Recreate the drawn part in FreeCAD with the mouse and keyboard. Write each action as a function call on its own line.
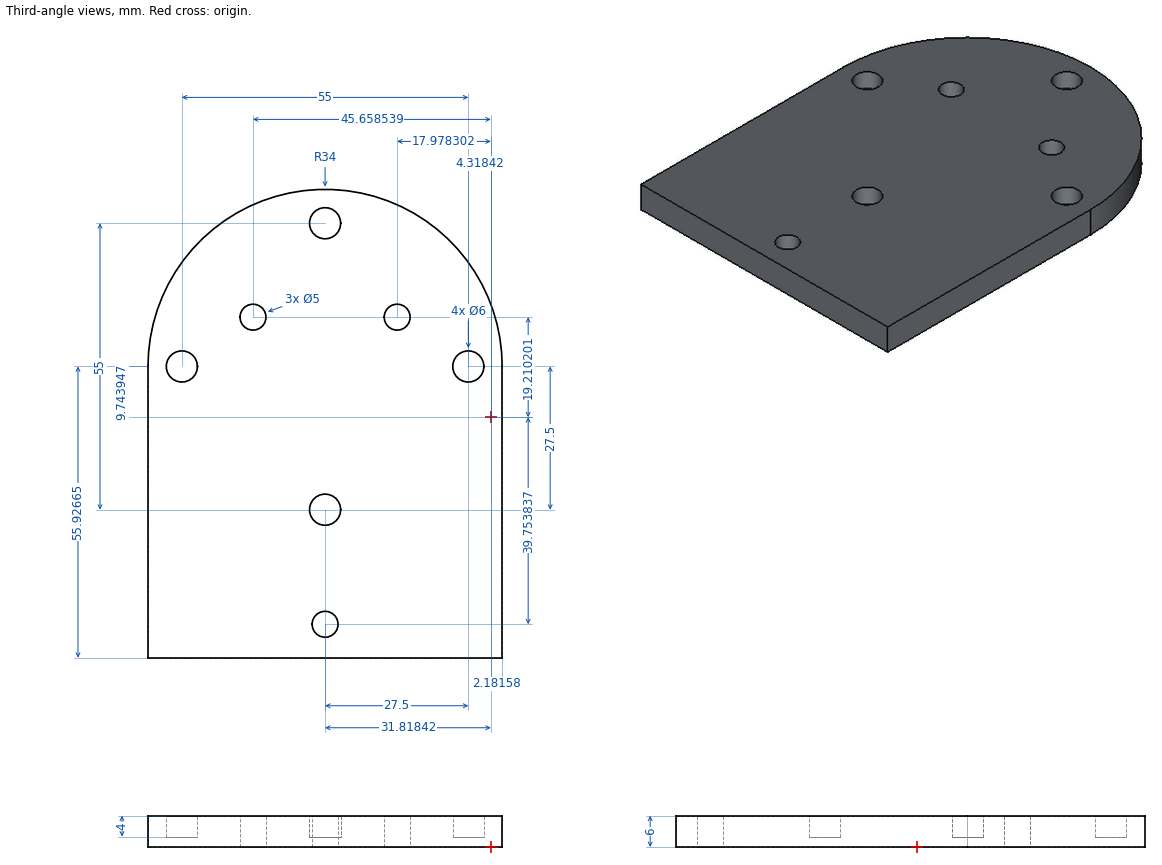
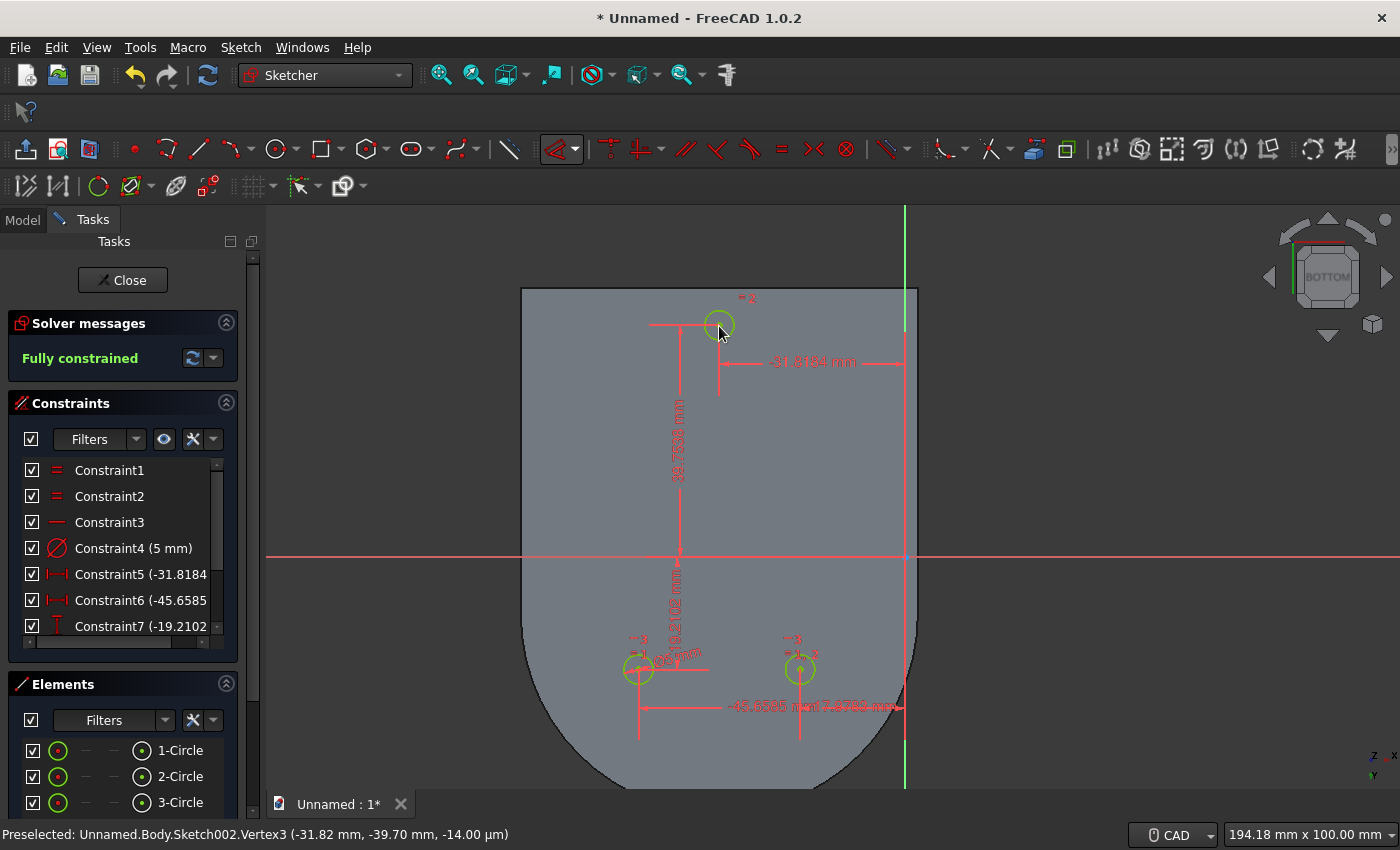
click(123, 280)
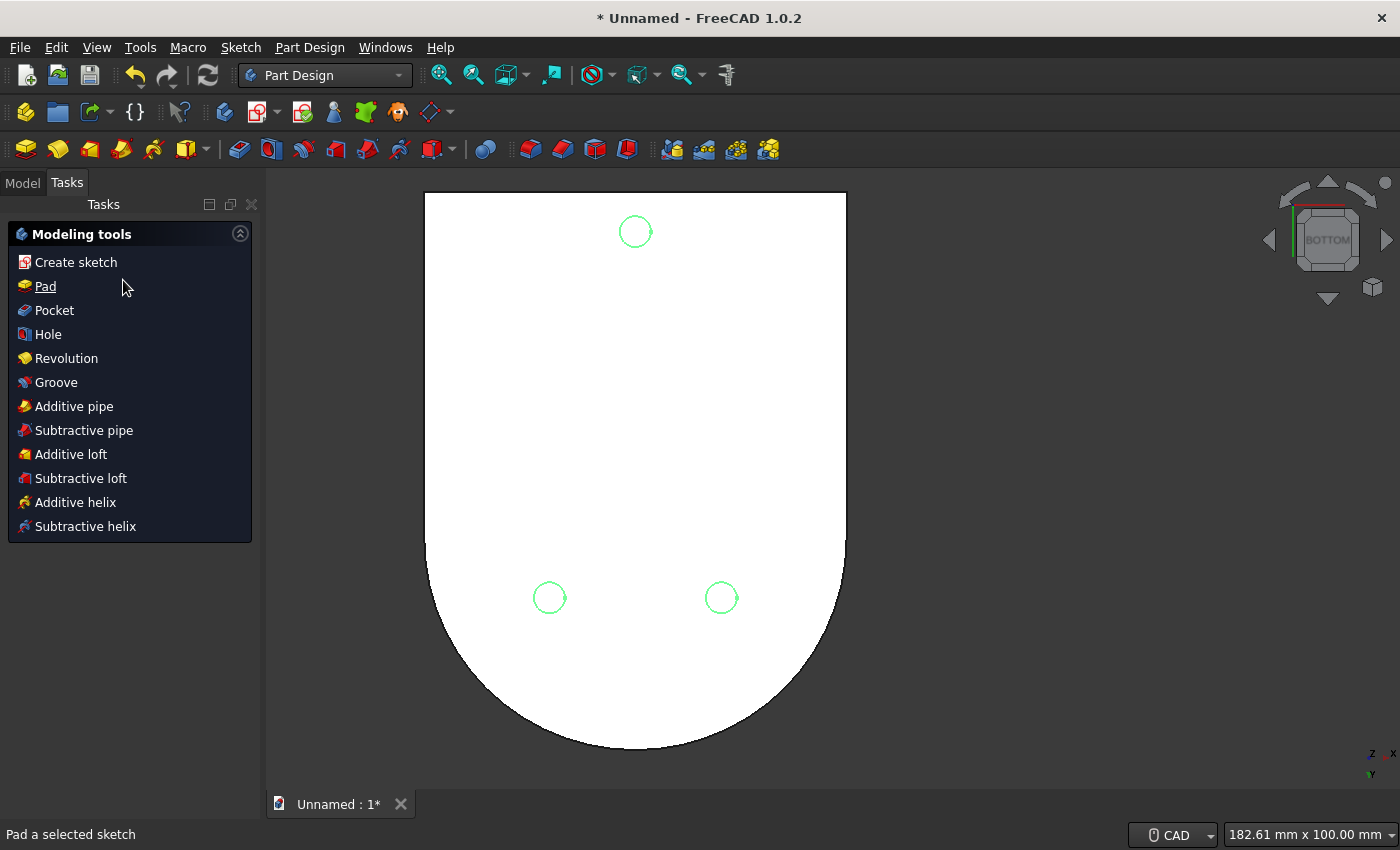
click(240, 150)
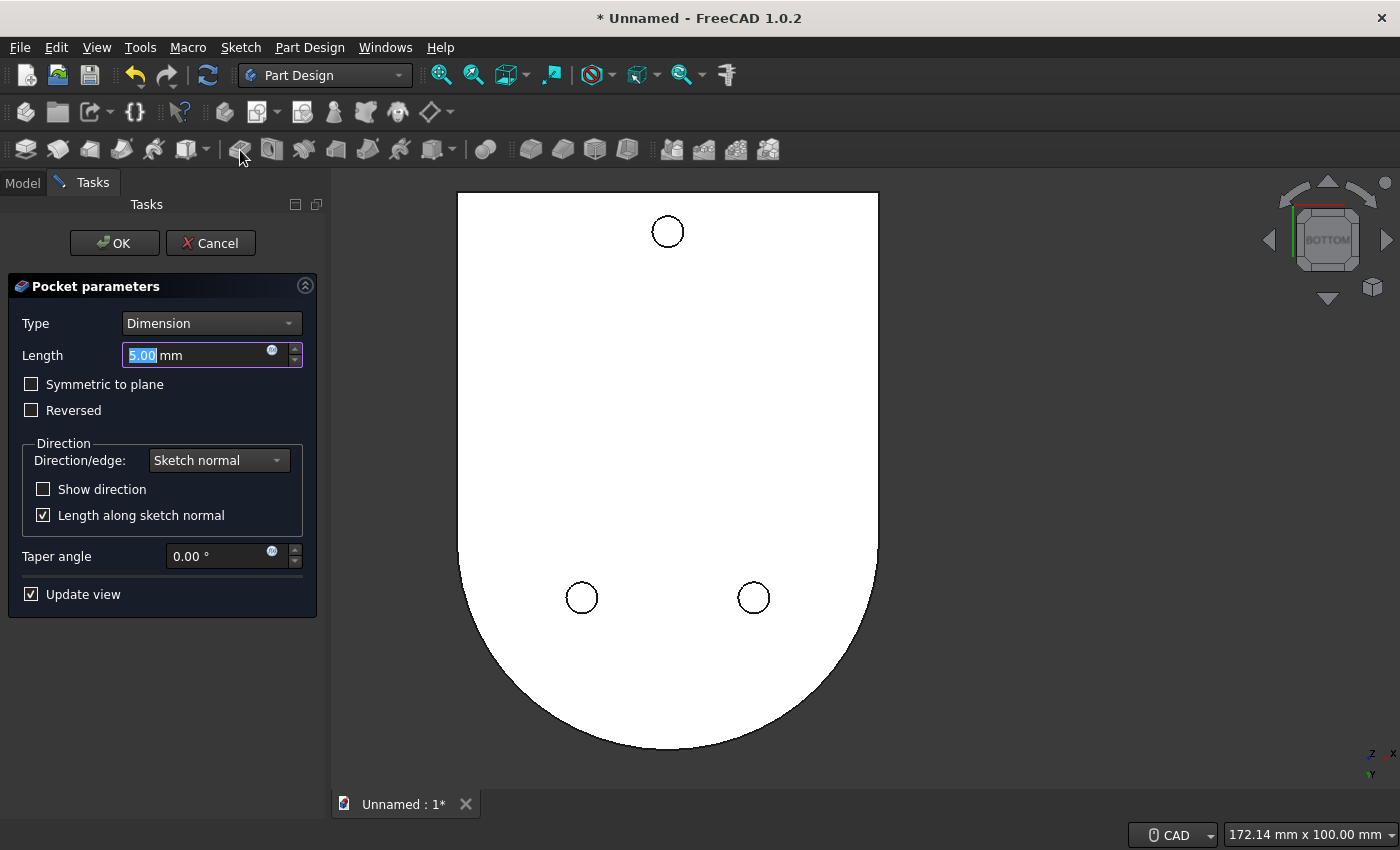
text(6)
key(Tab)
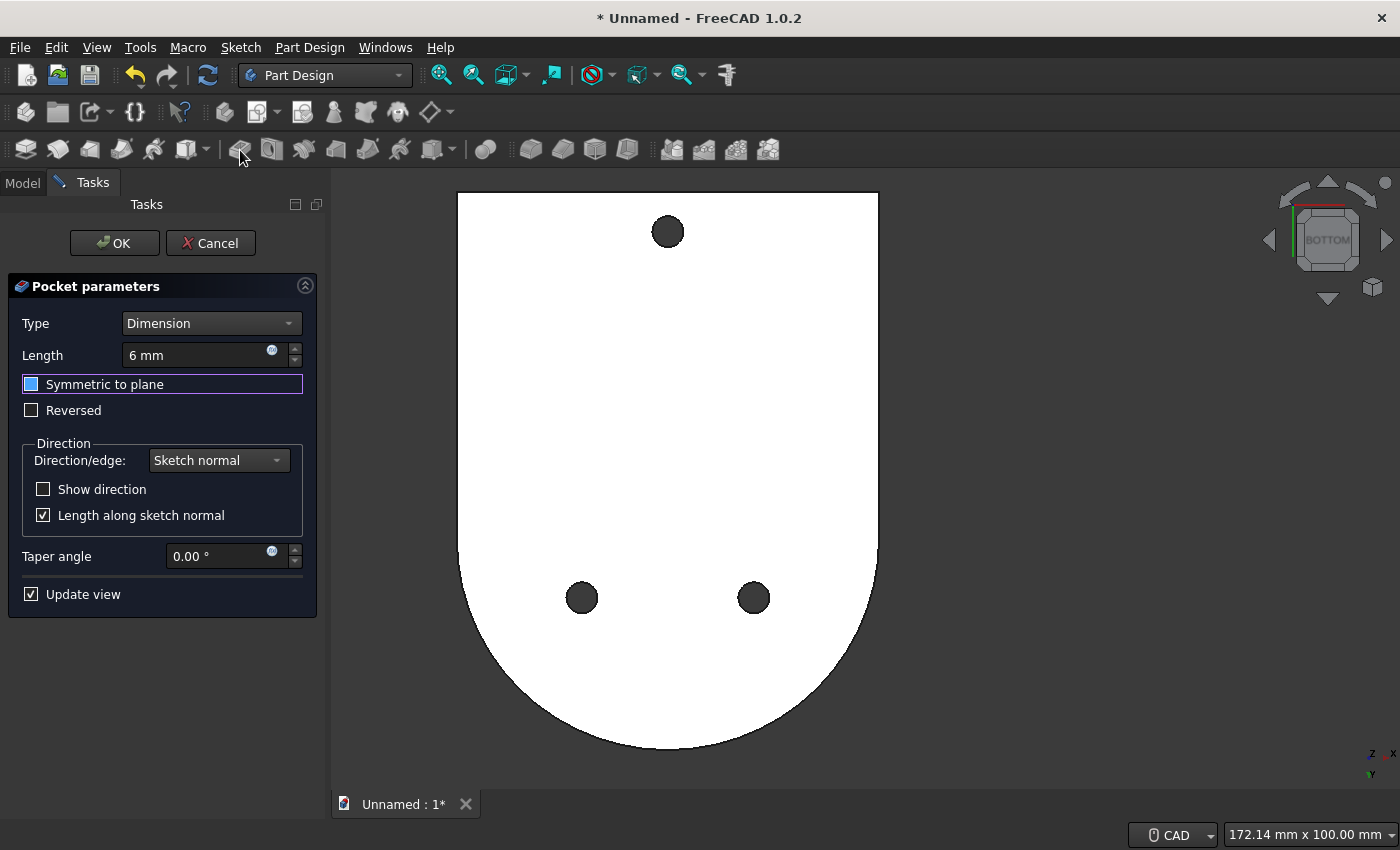
click(115, 243)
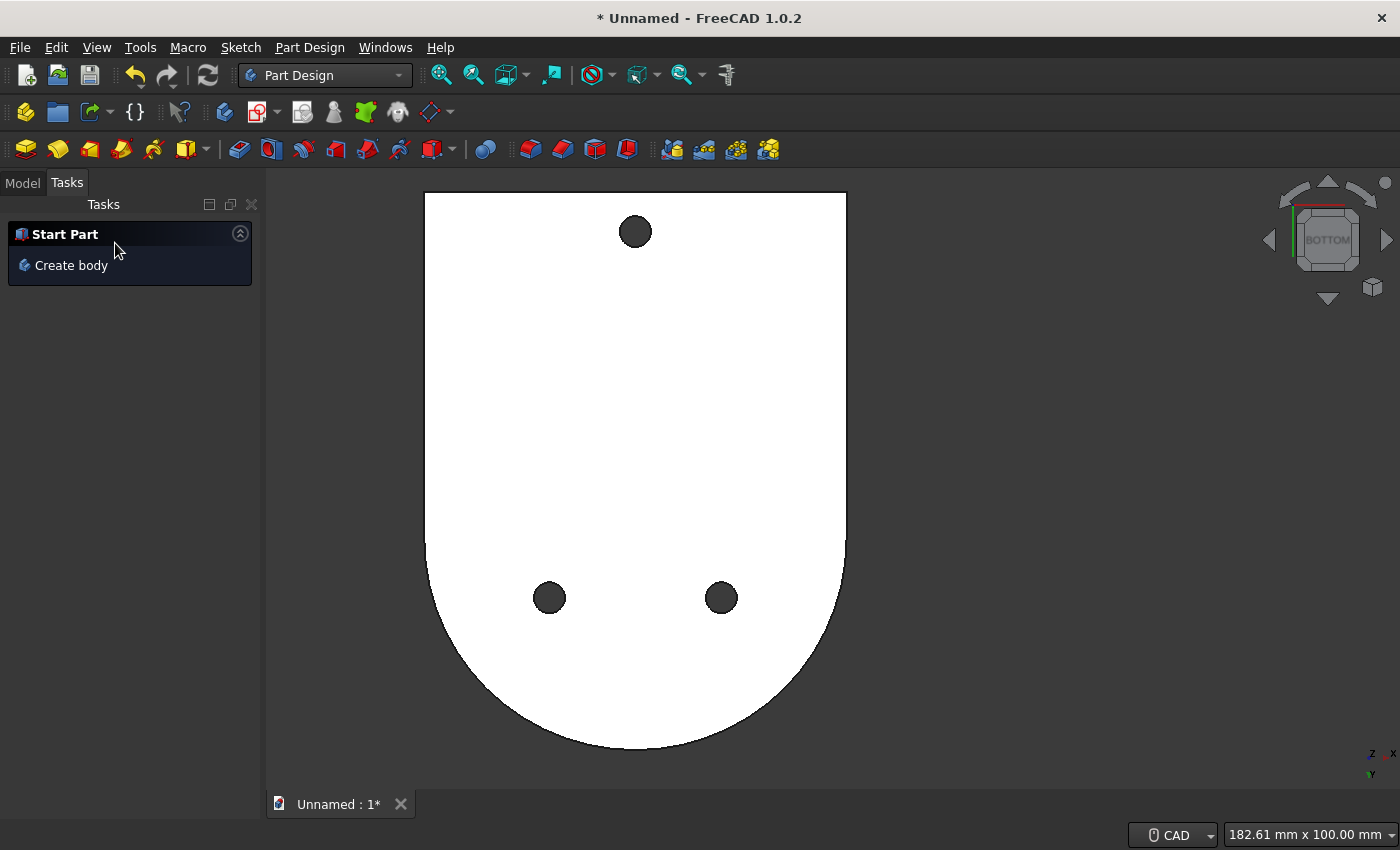
key(0)